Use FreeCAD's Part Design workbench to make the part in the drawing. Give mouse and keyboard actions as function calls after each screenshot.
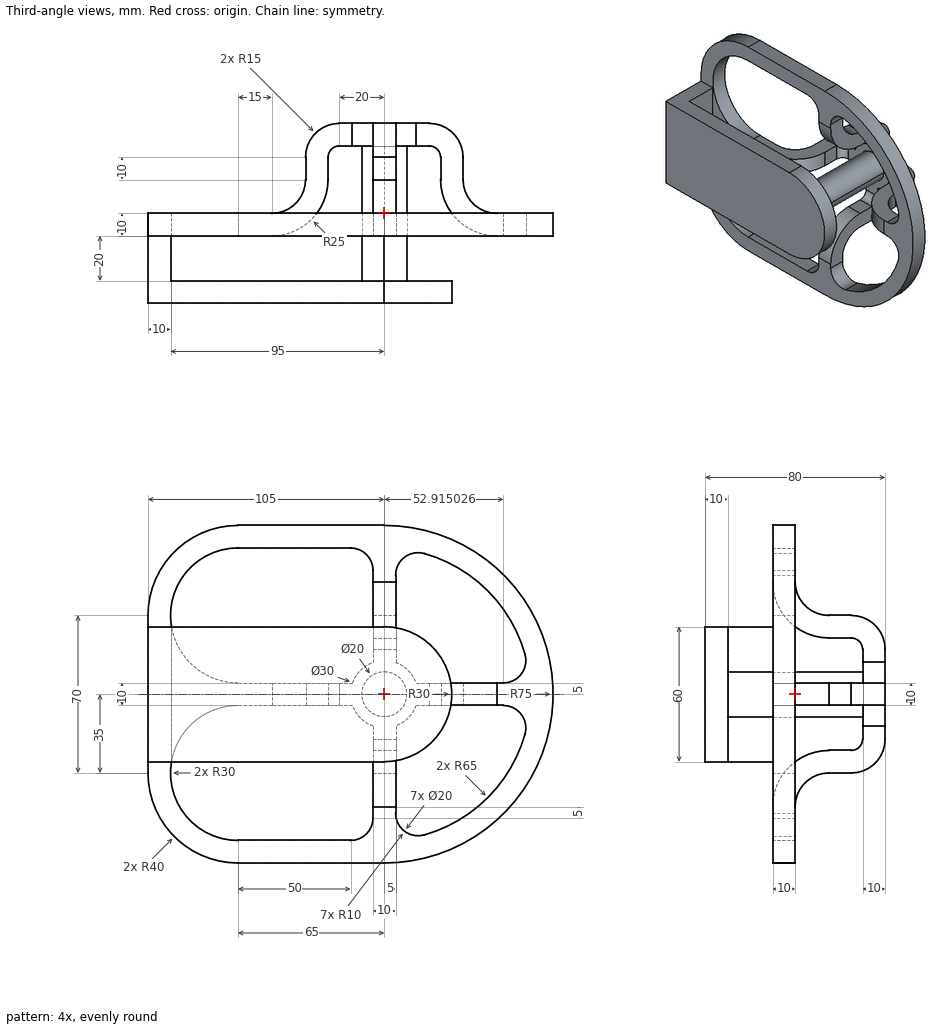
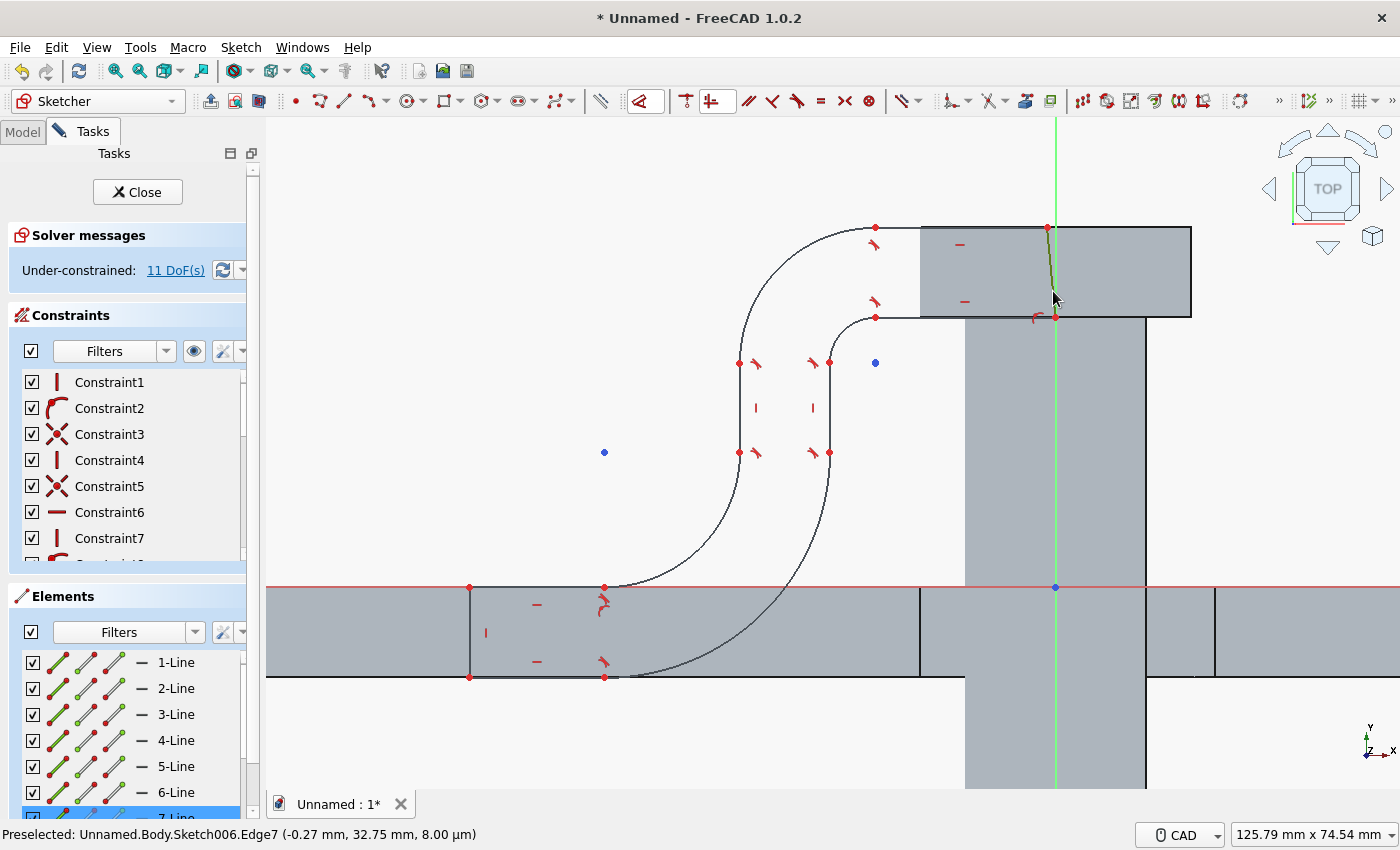
click(730, 102)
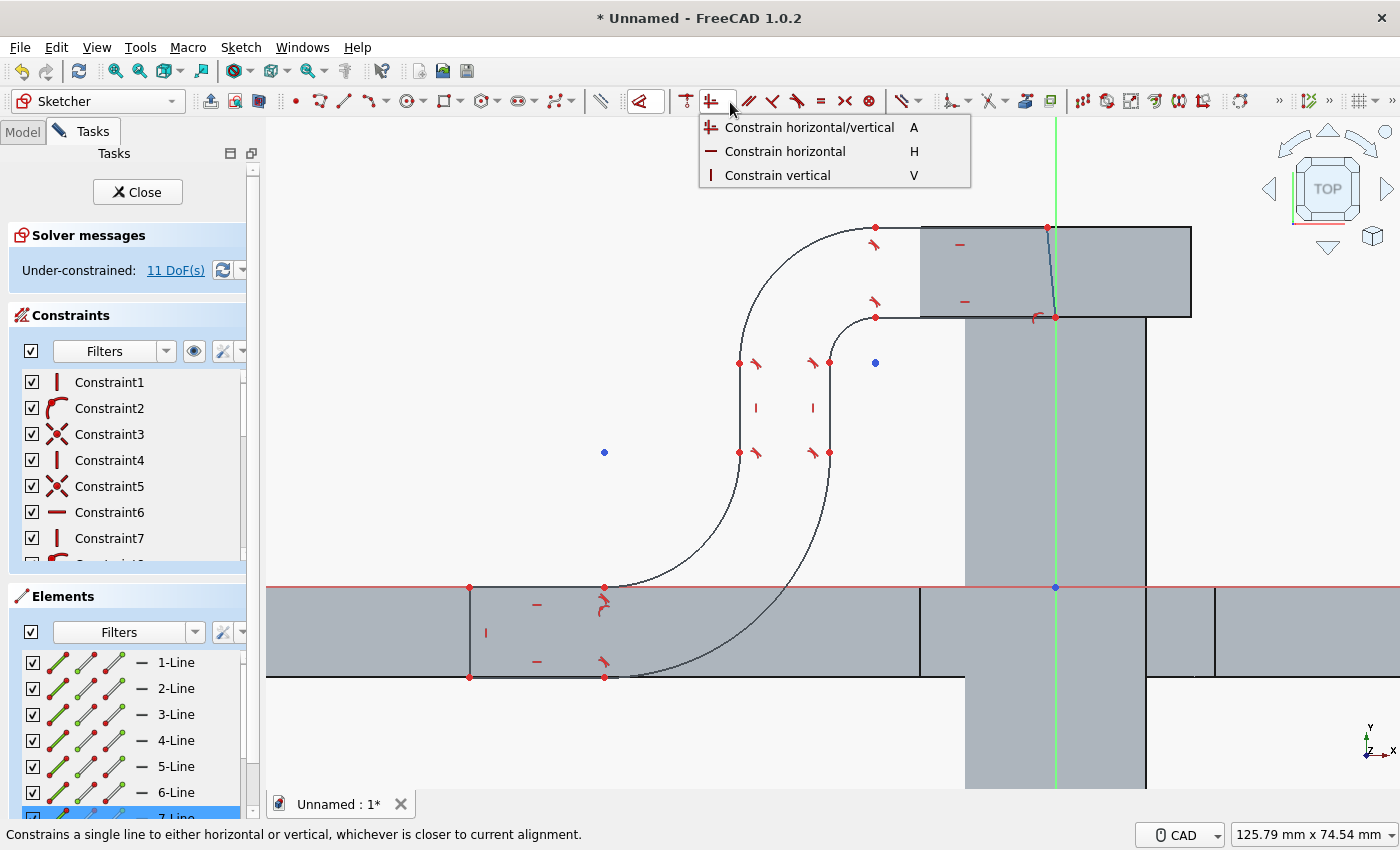
click(835, 175)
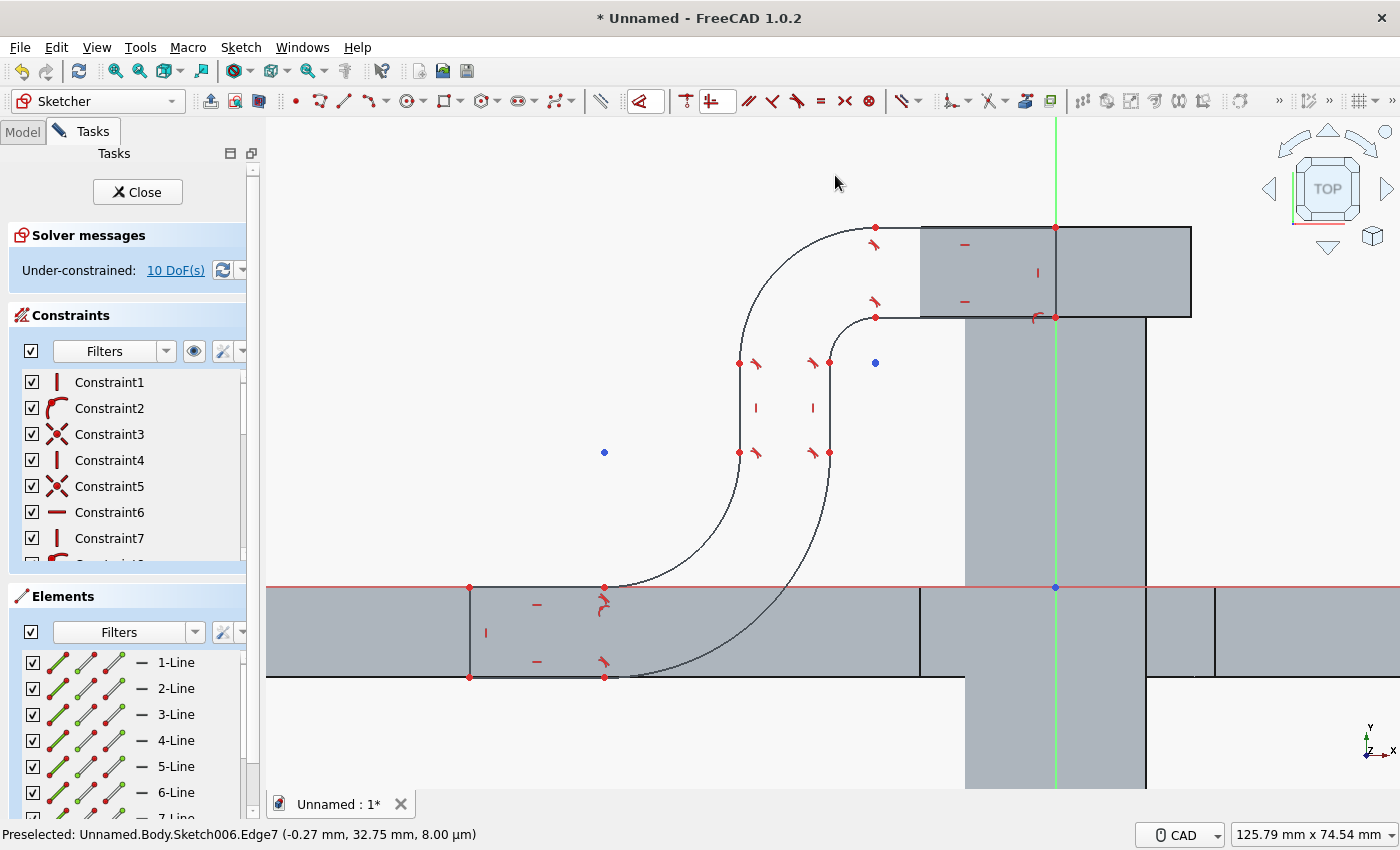
click(666, 573)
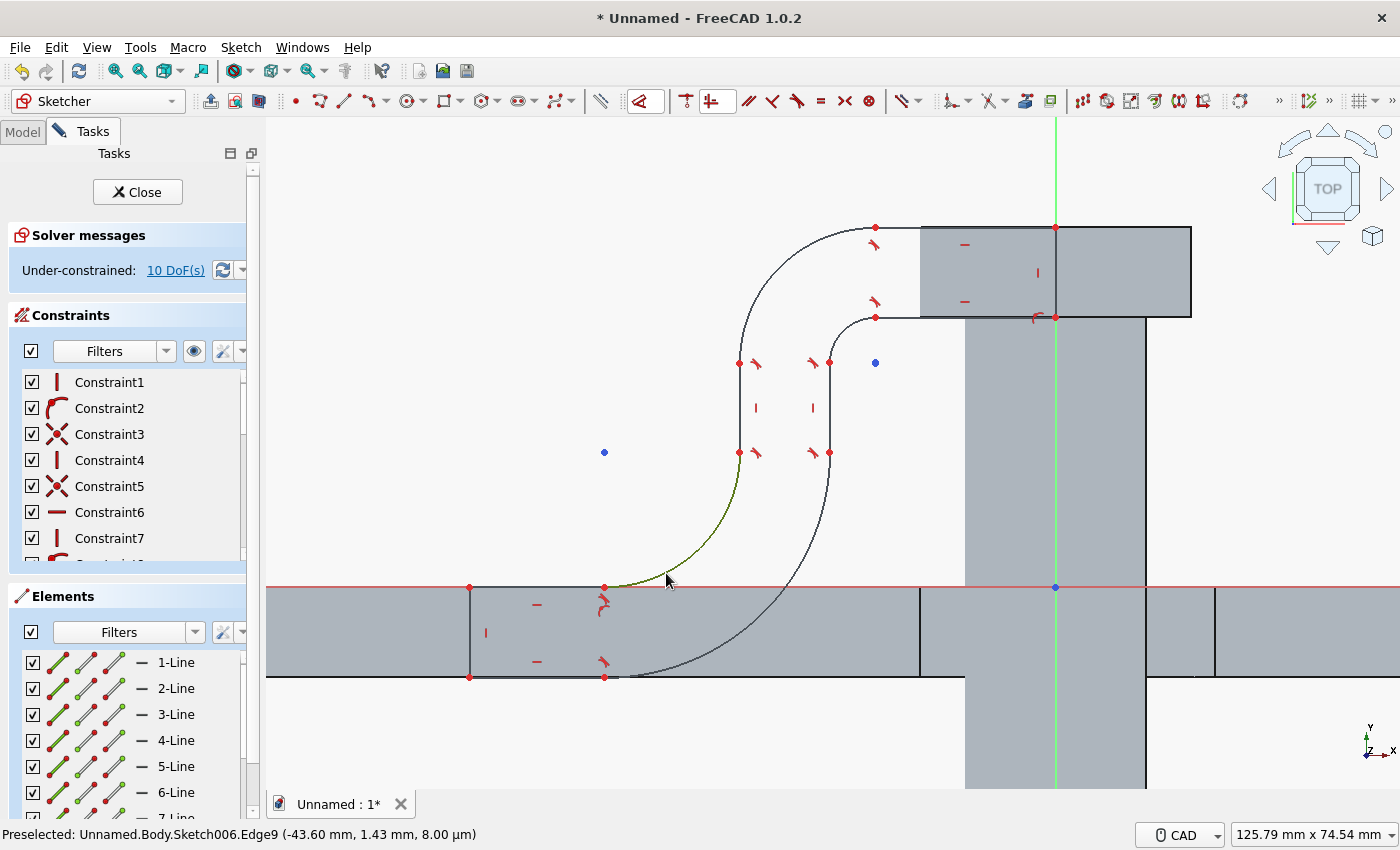
click(707, 653)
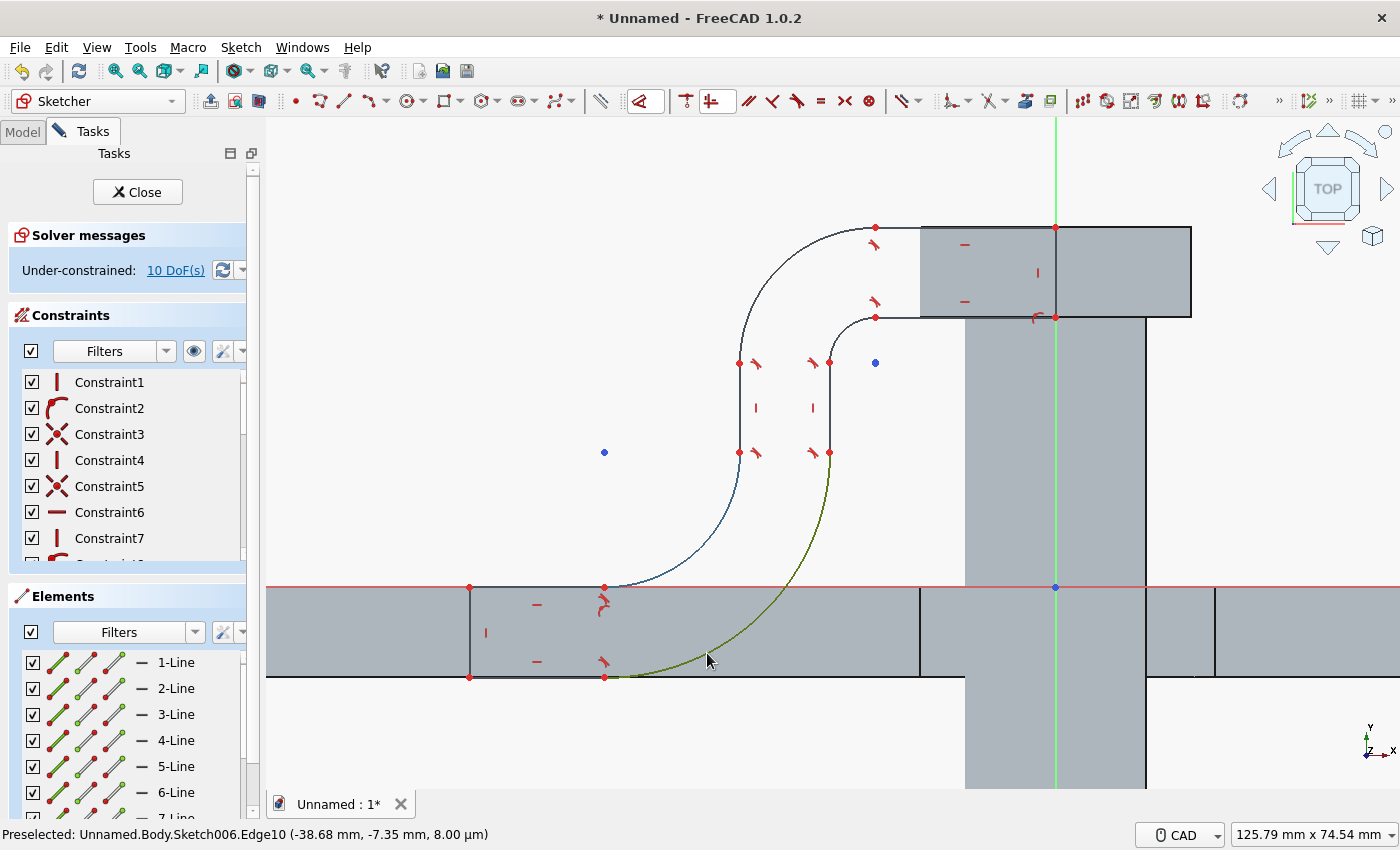
click(686, 102)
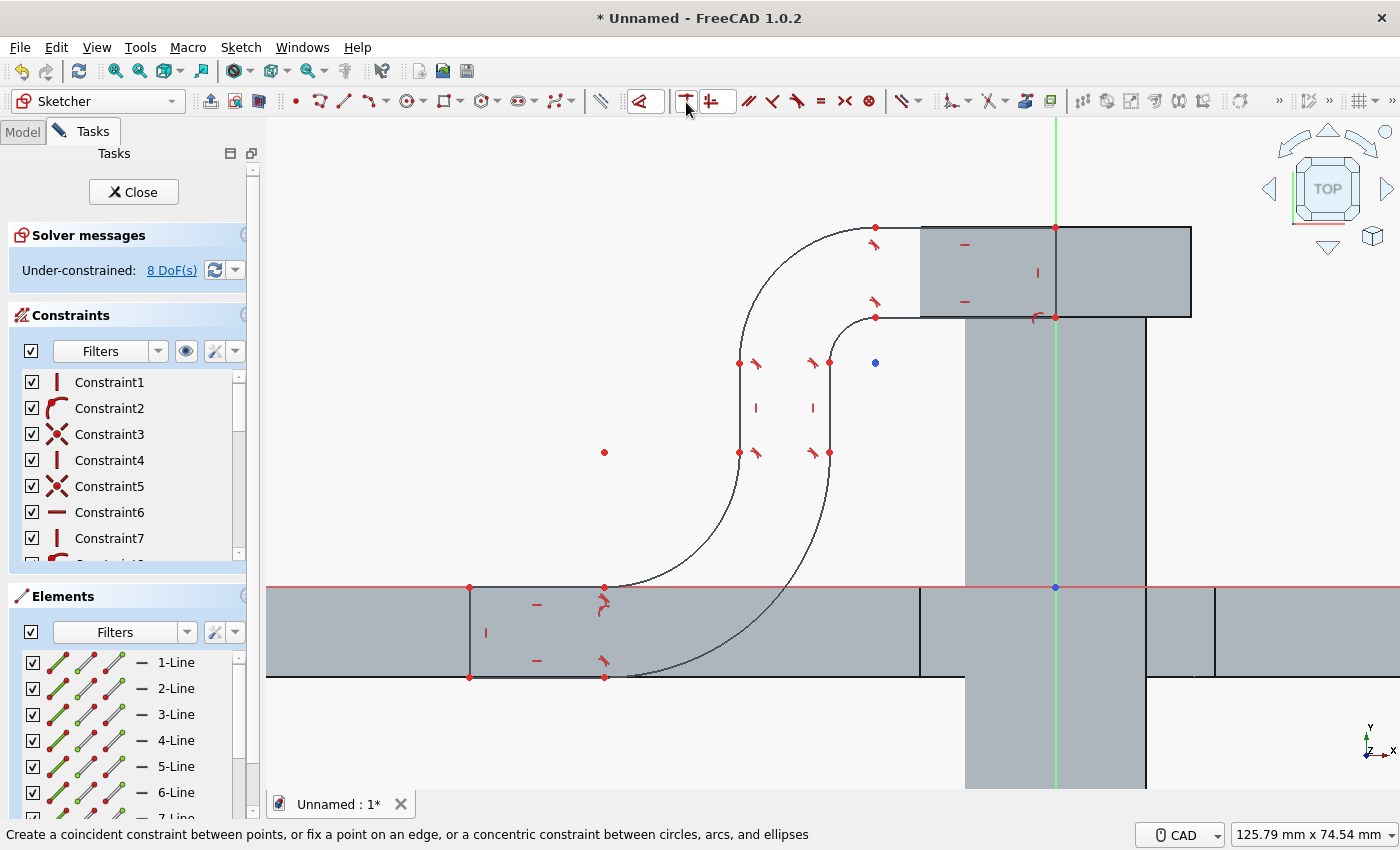
click(855, 323)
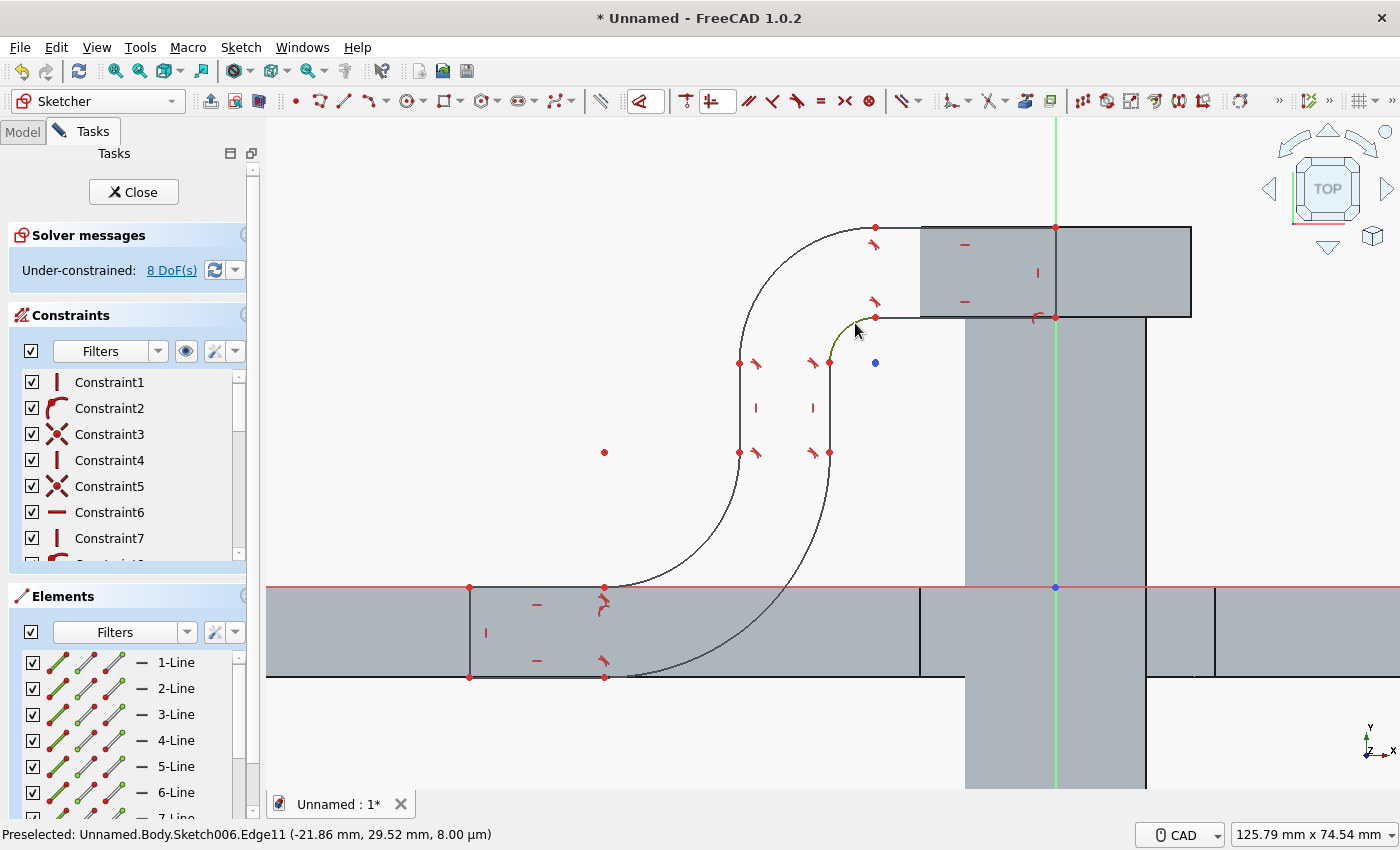
click(814, 242)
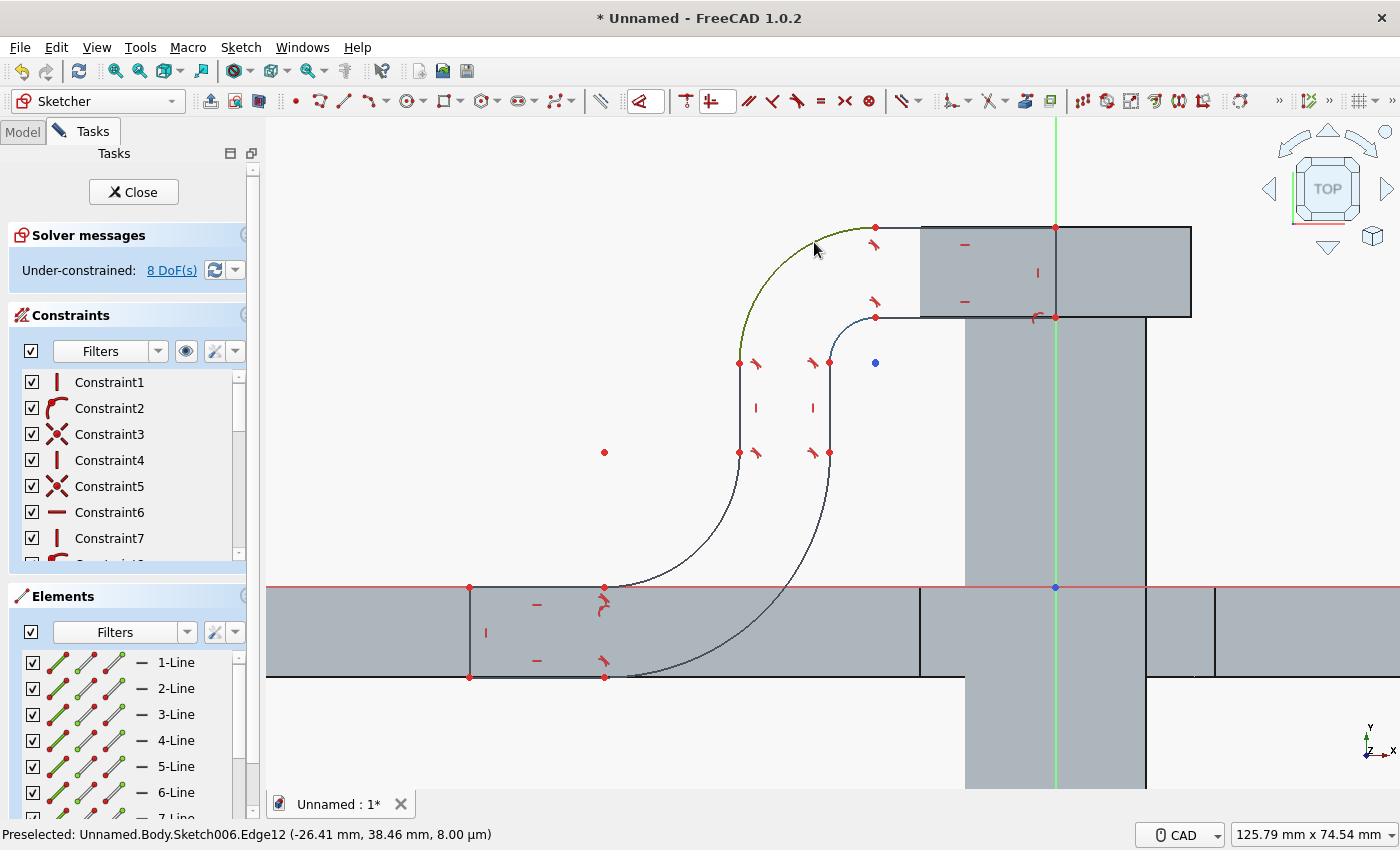
click(686, 102)